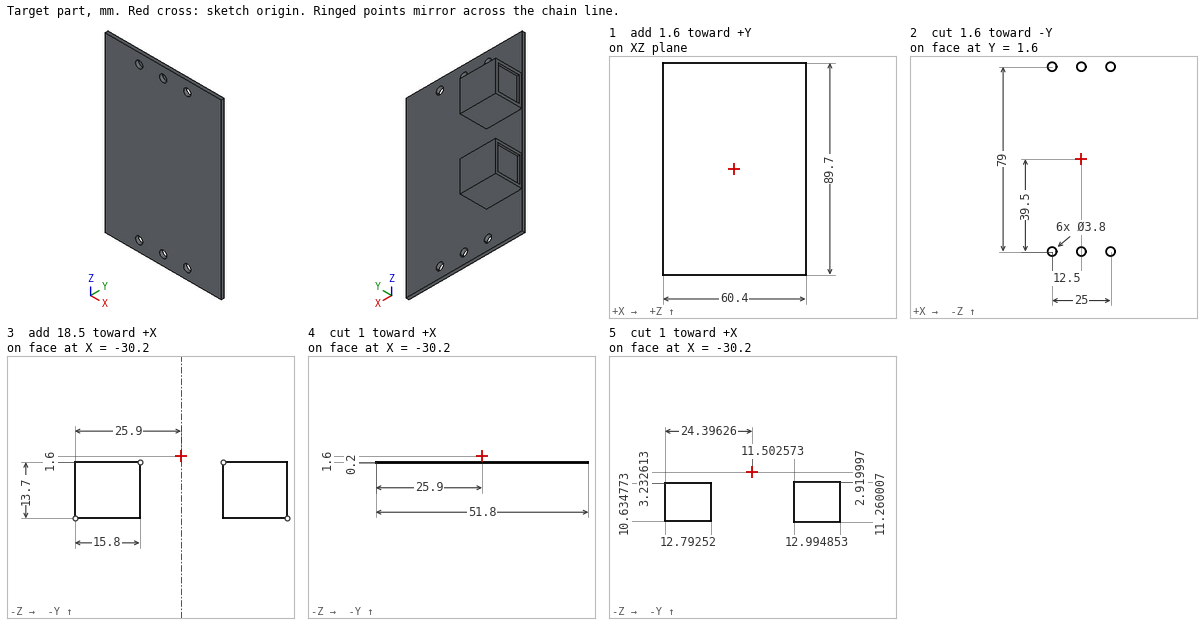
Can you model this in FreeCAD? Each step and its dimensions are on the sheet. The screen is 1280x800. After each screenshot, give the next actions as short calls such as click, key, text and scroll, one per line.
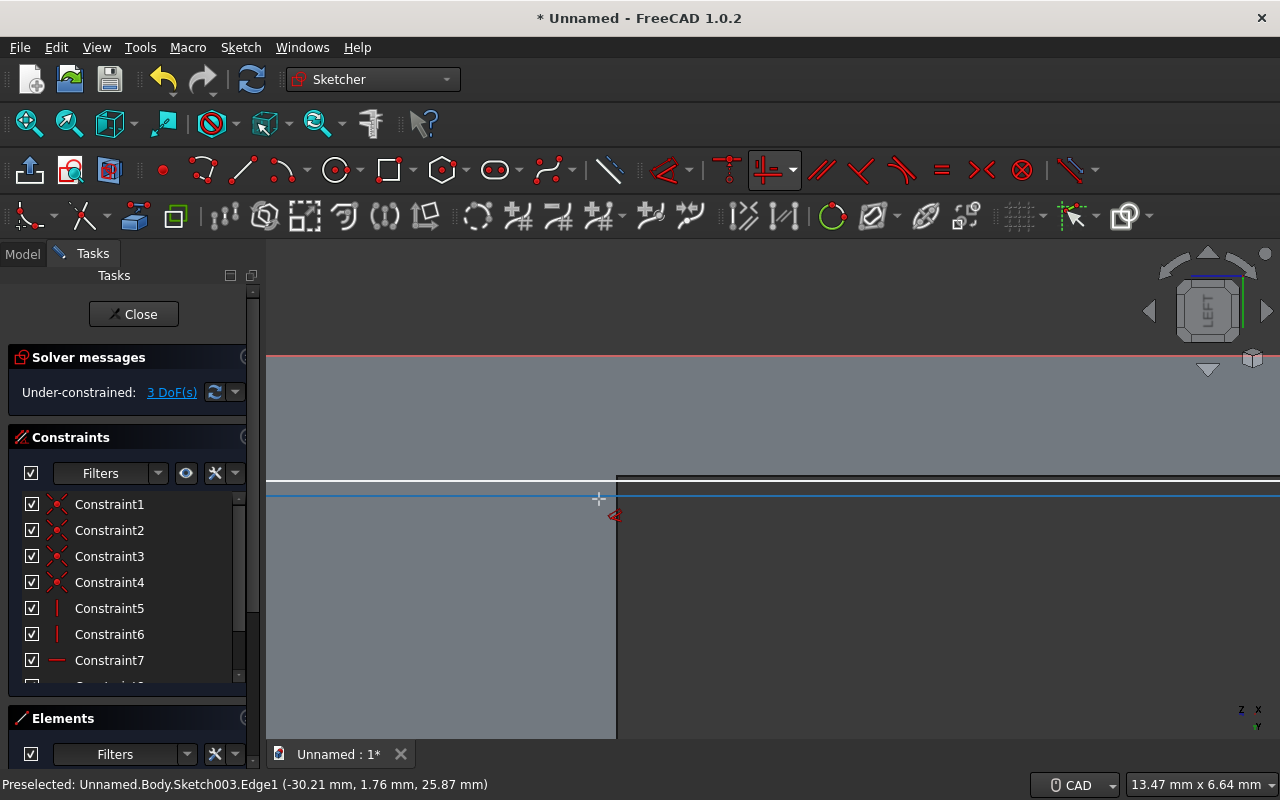
click(598, 496)
click(704, 530)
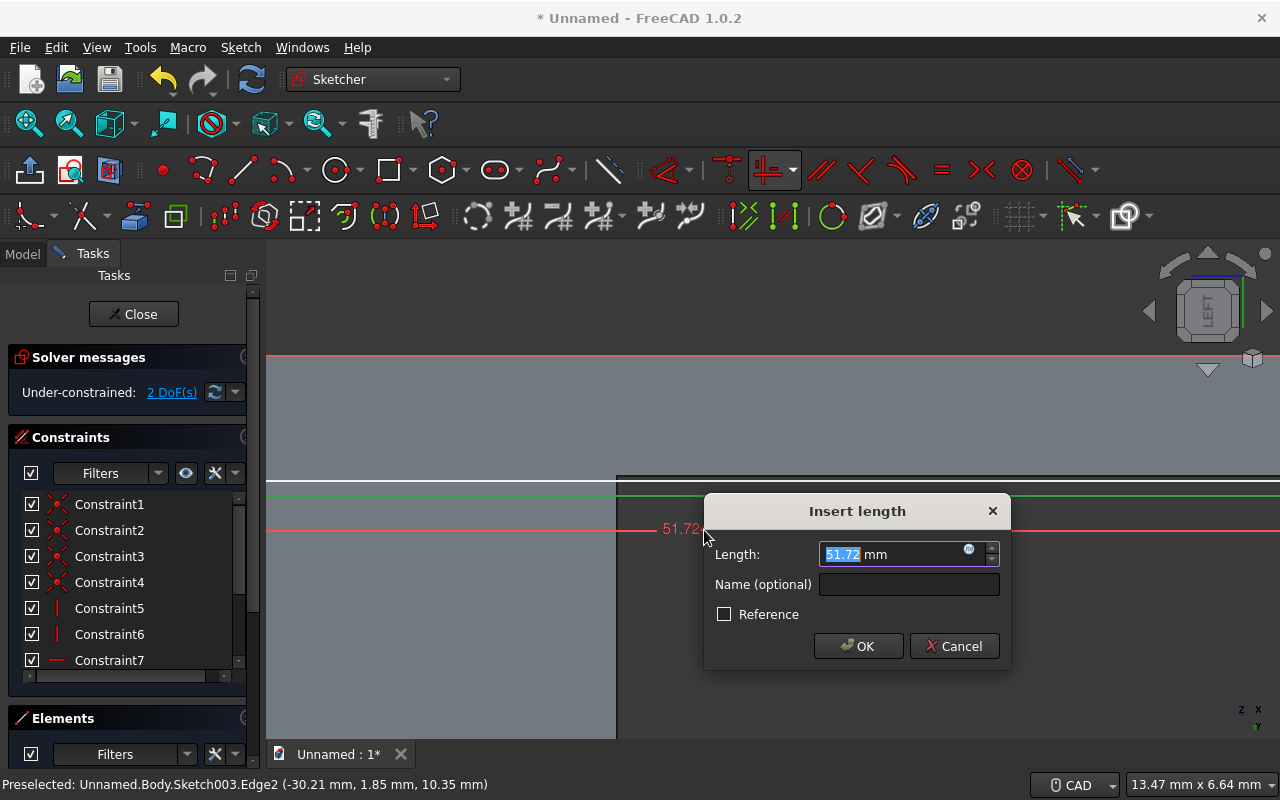
text(51.8)
key(Return)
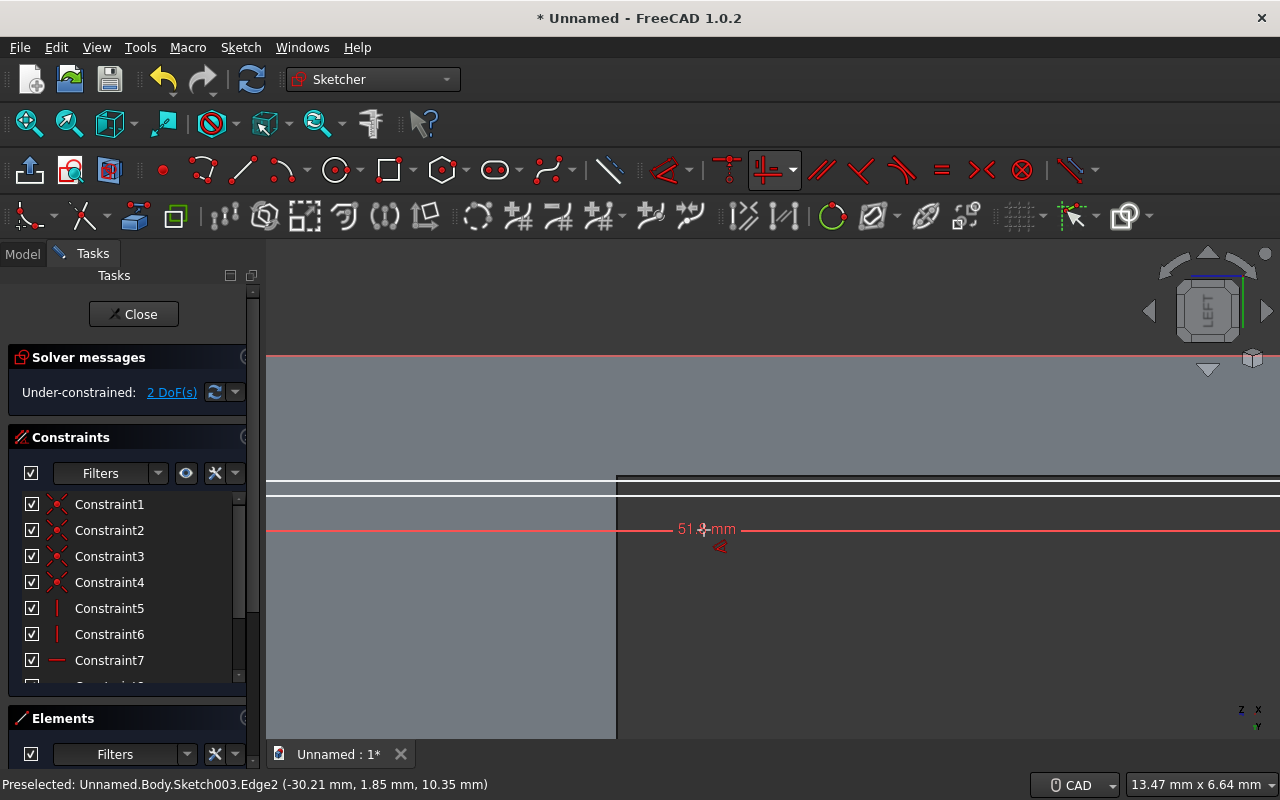
scroll(599, 499, down, 10)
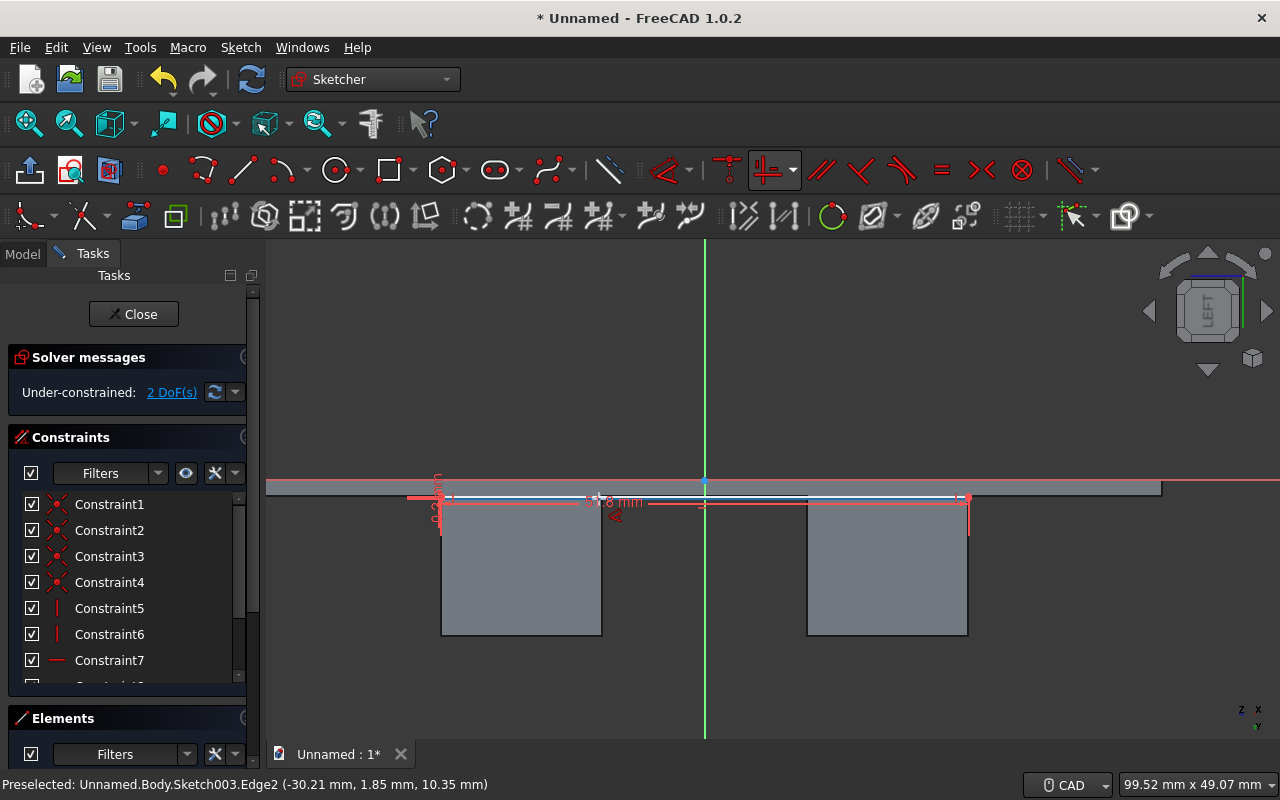
scroll(441, 497, up, 9)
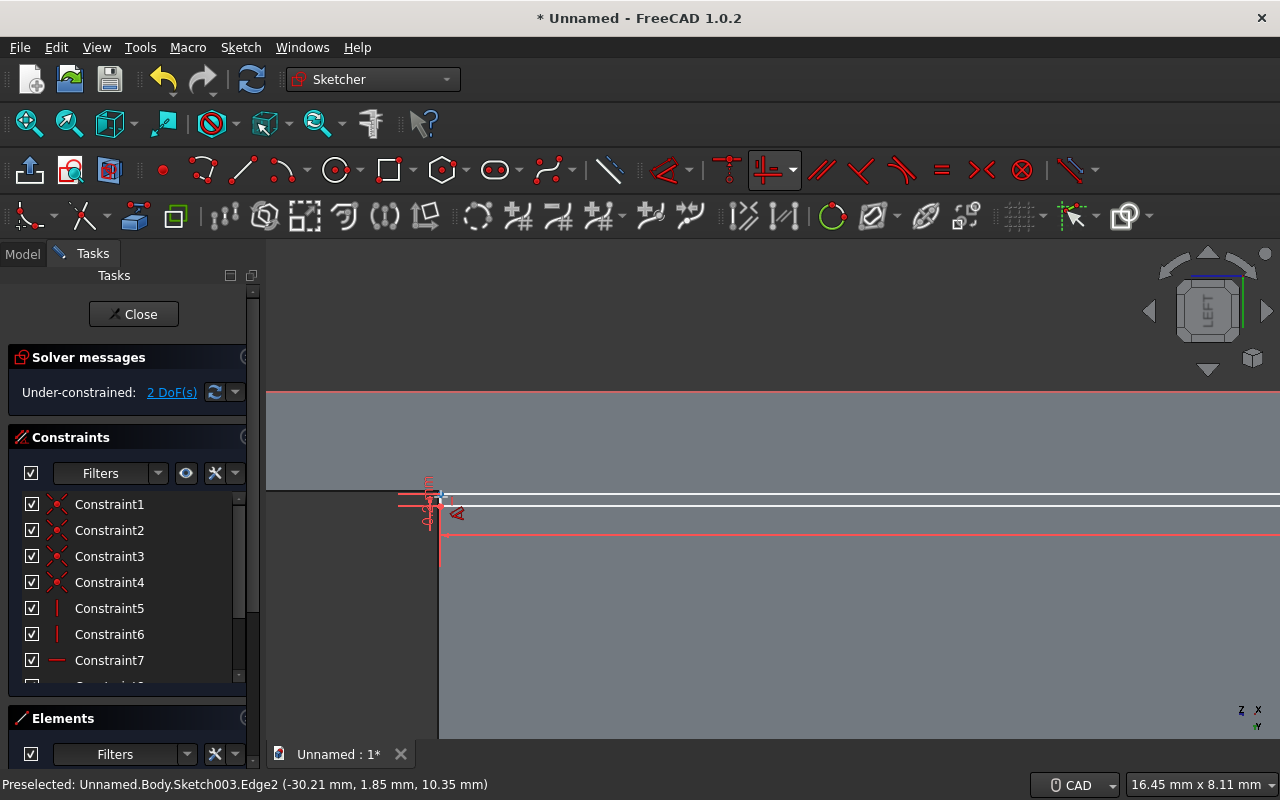
click(440, 494)
click(406, 443)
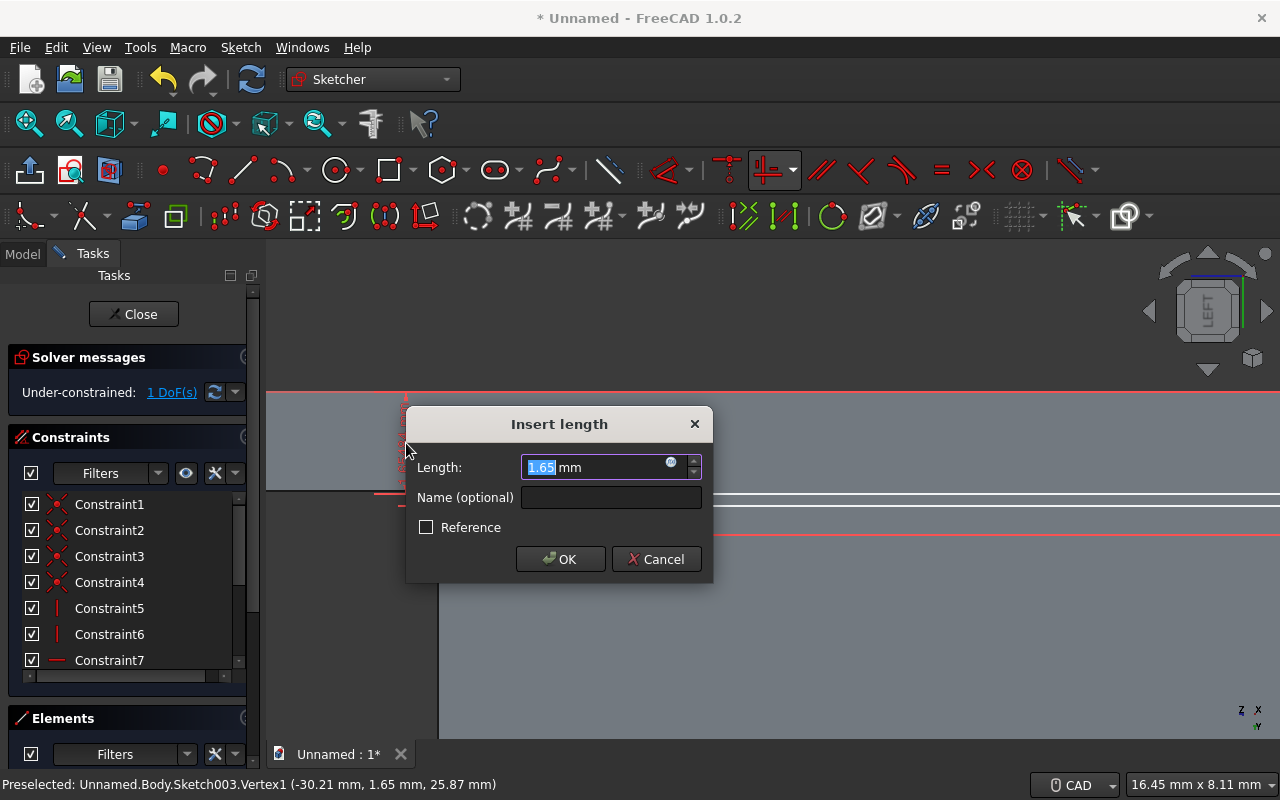
text(1.6)
key(Return)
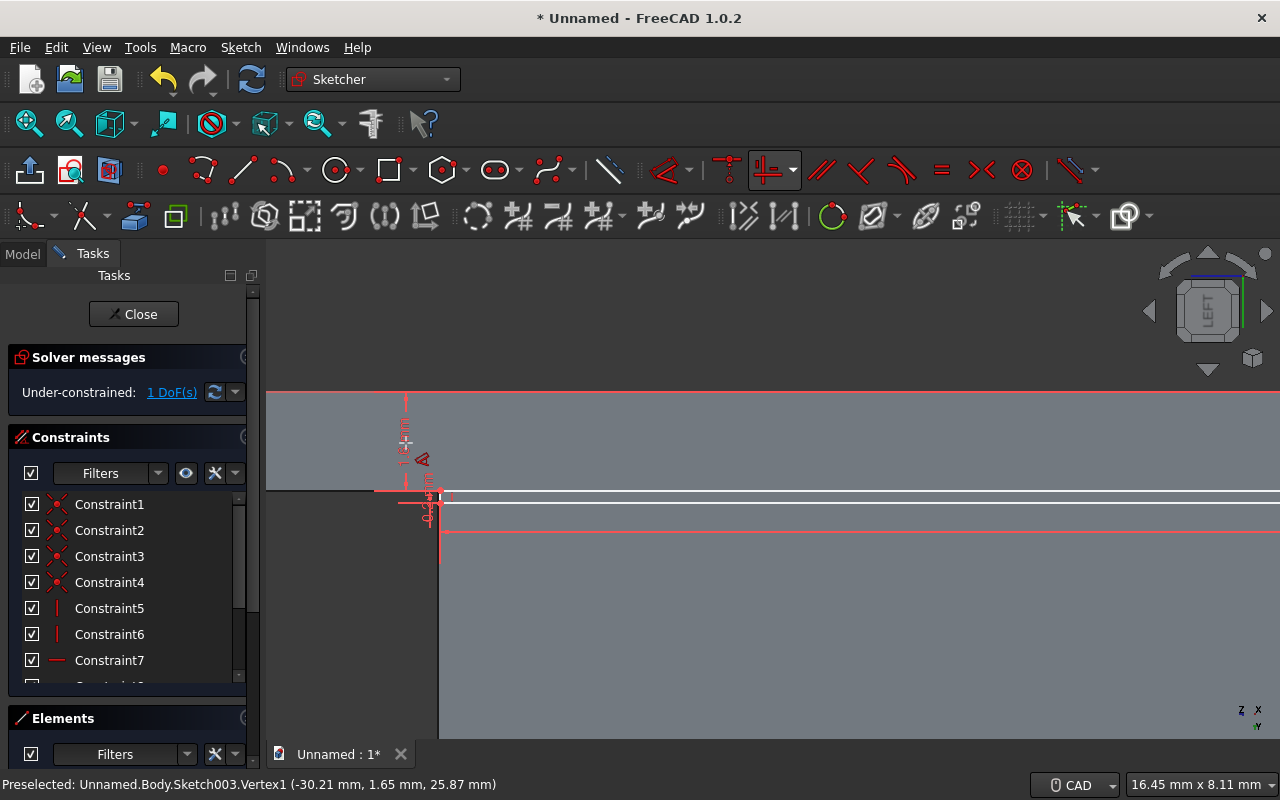
click(440, 491)
click(778, 358)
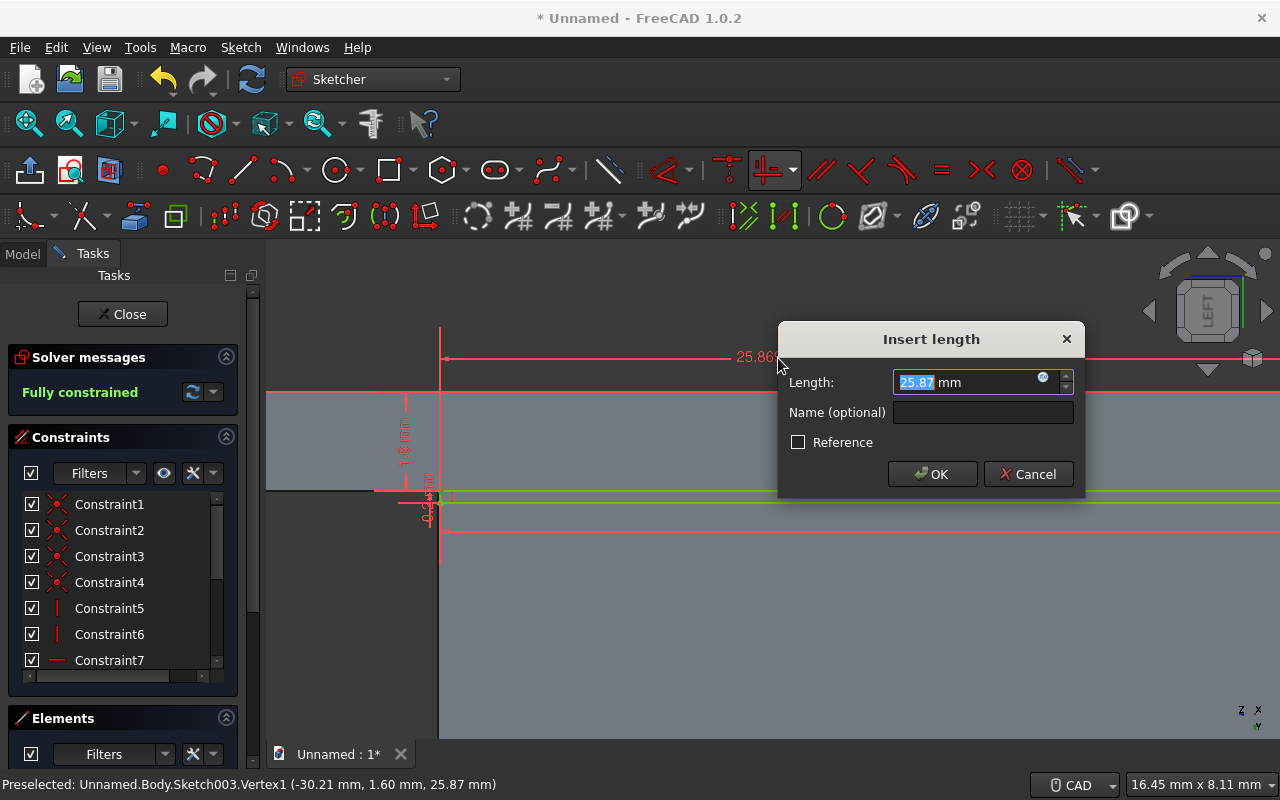
text(25.9)
key(Return)
key(Escape)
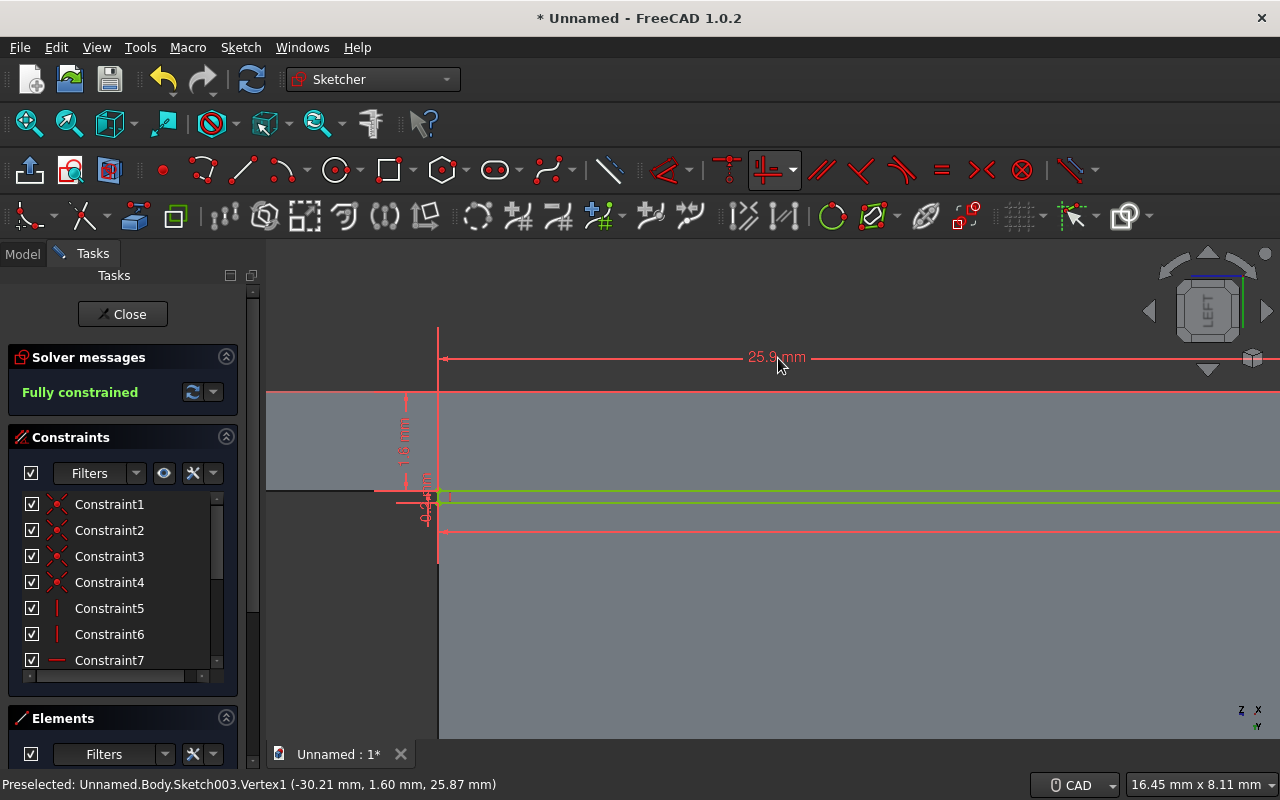
click(123, 314)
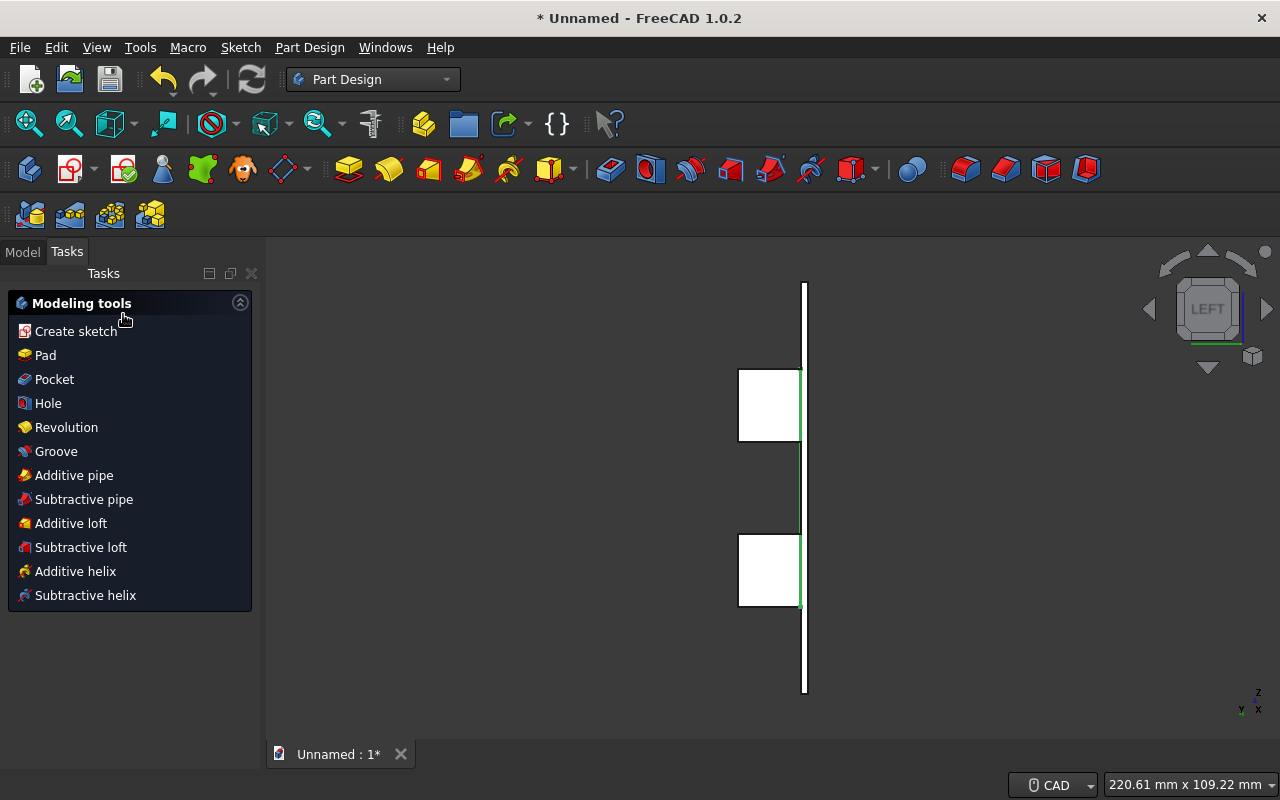
click(612, 170)